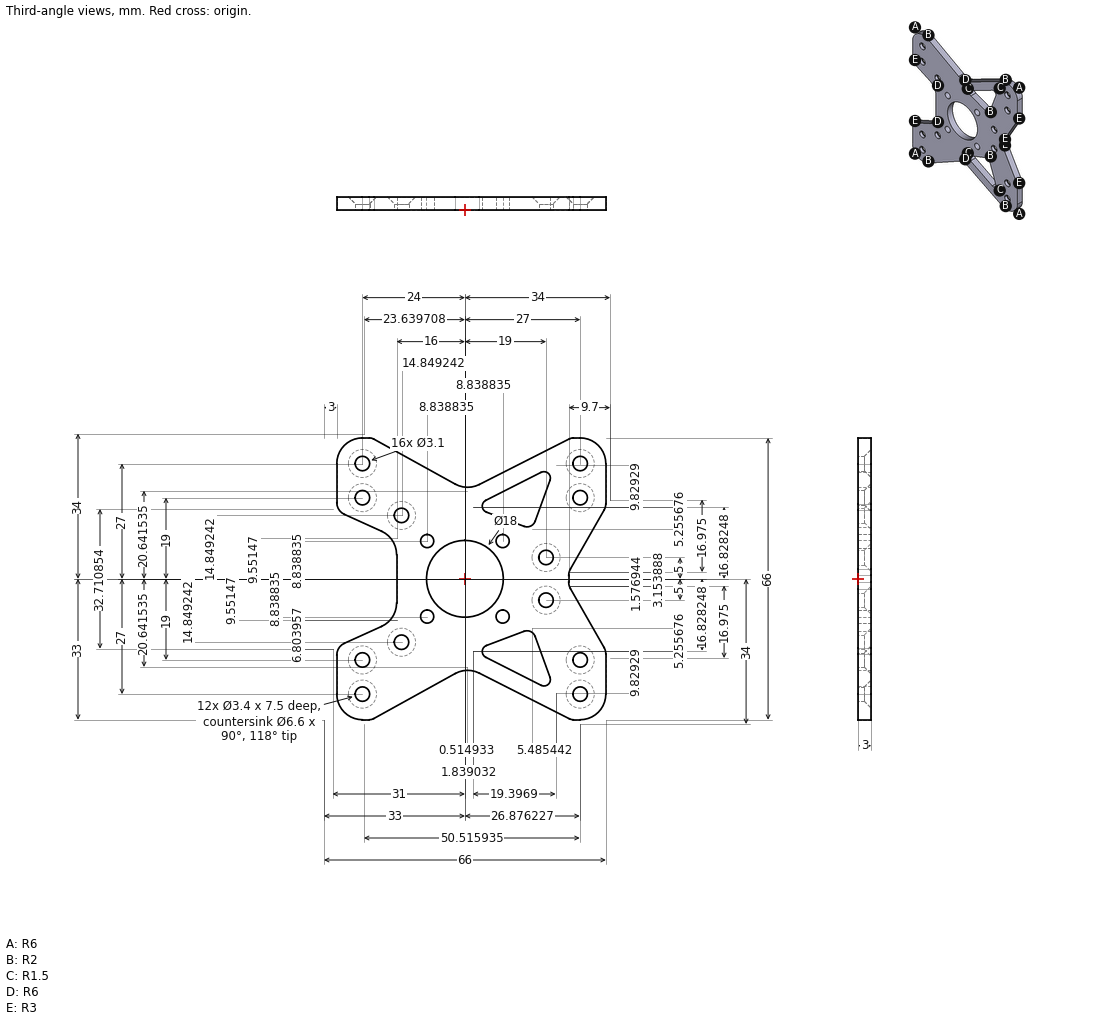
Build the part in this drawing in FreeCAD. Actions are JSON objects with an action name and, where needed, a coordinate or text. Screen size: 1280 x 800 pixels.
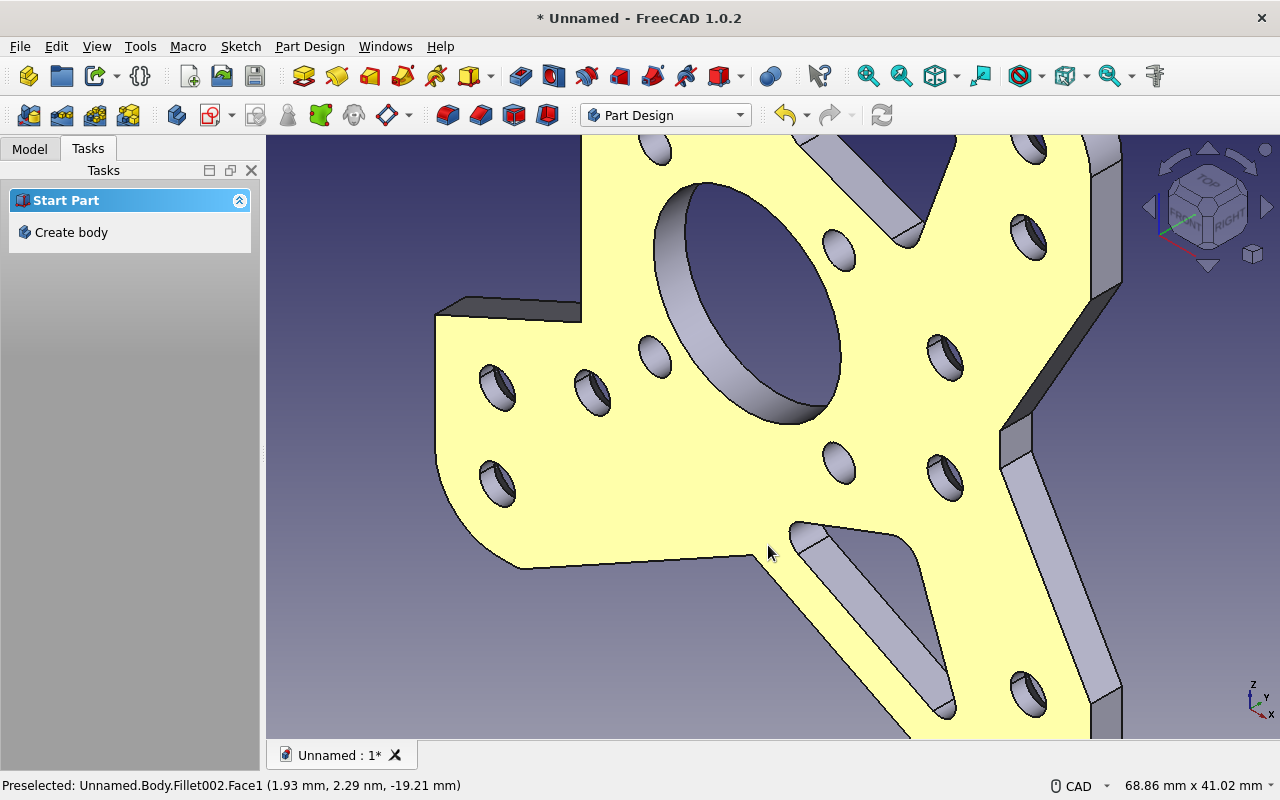
{"action": "left_click", "coordinate": [869, 76]}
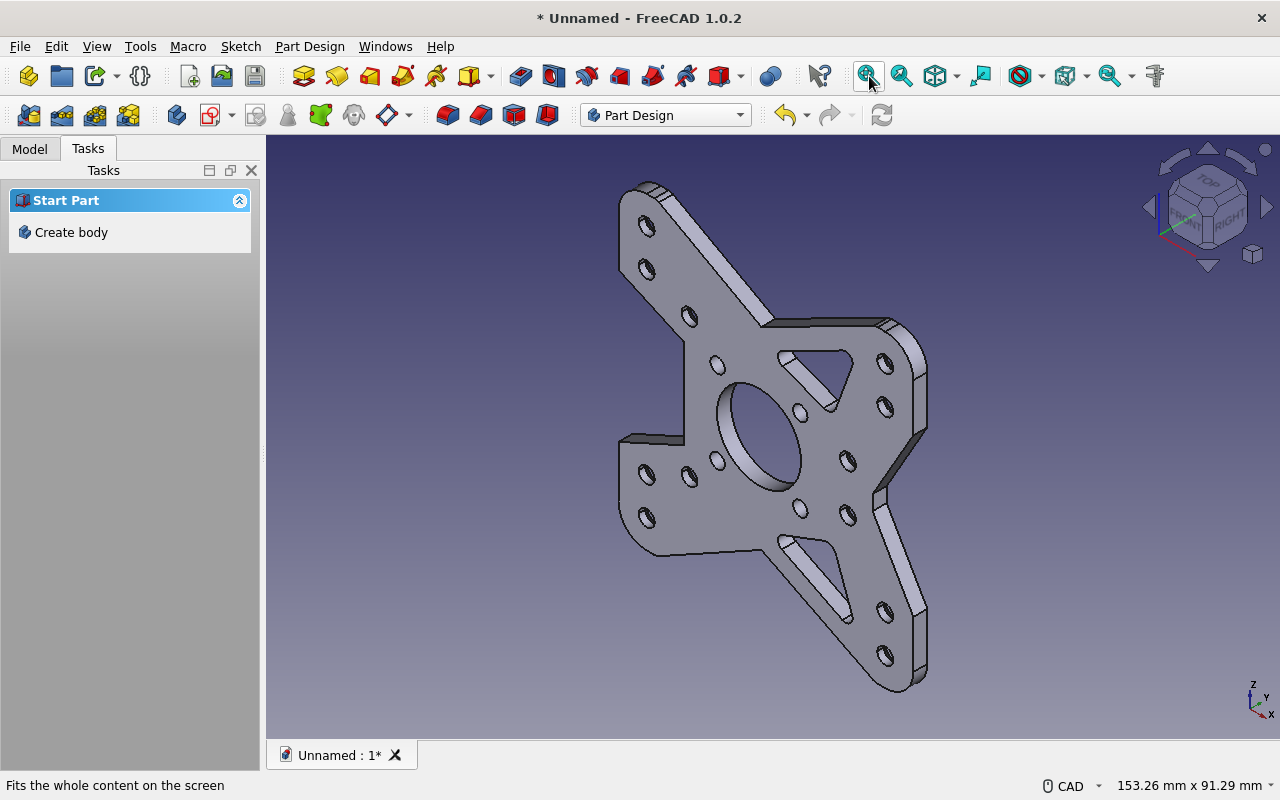
{"action": "key", "text": "2"}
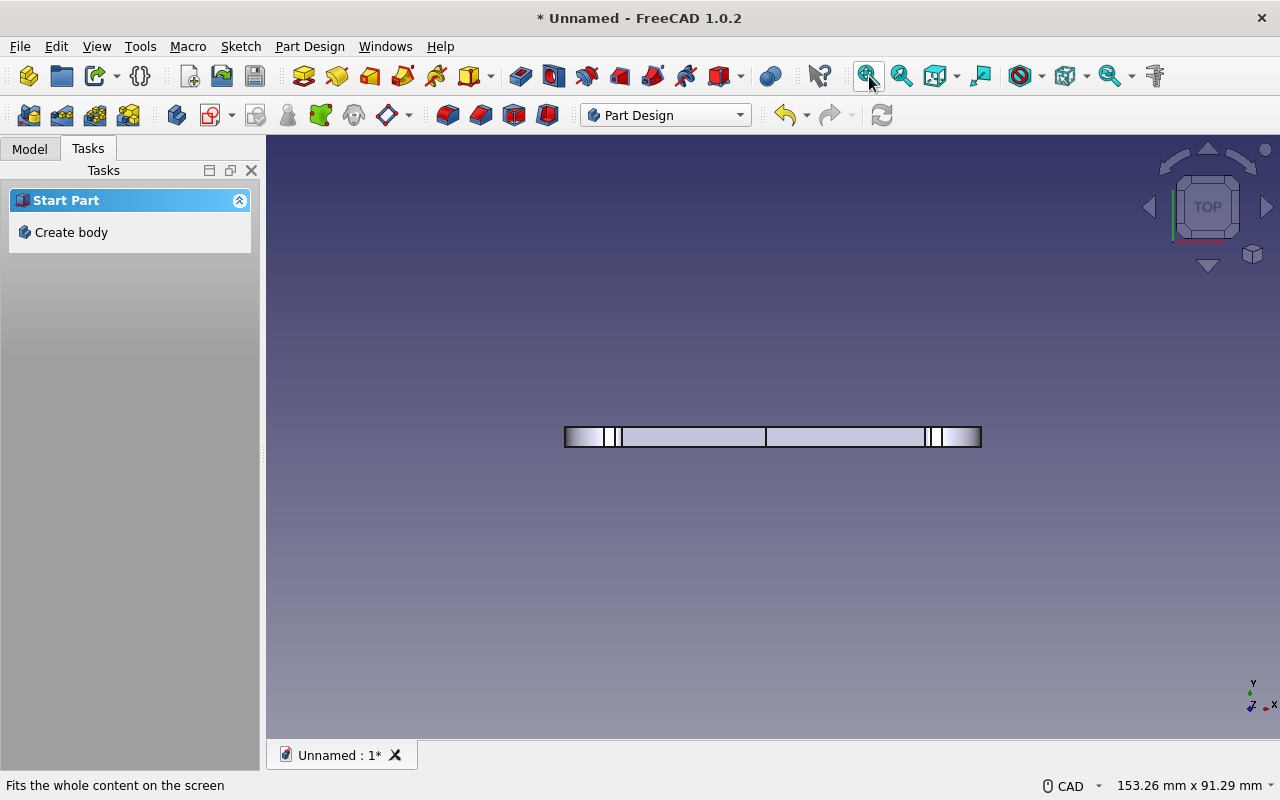
{"action": "key", "text": "v f"}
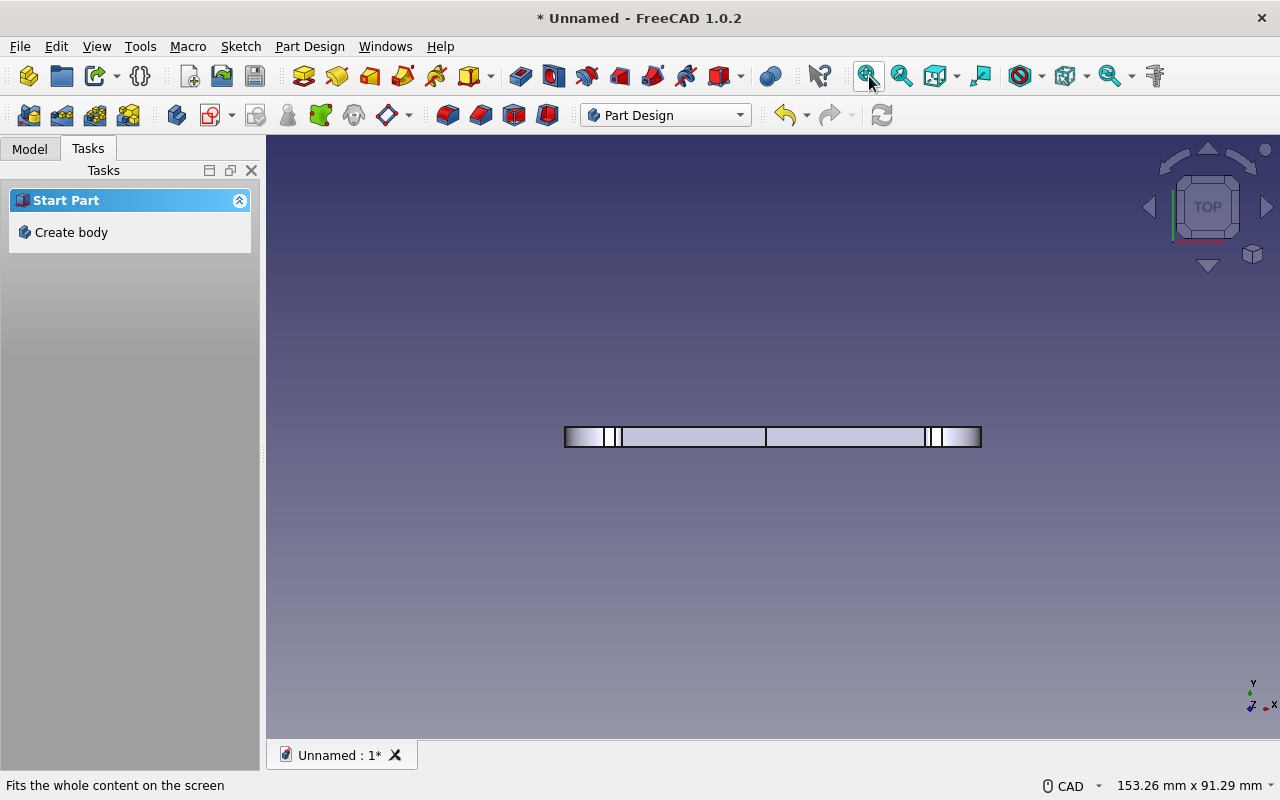
{"action": "scroll", "coordinate": [766, 436], "scroll_direction": "up", "scroll_amount": 4}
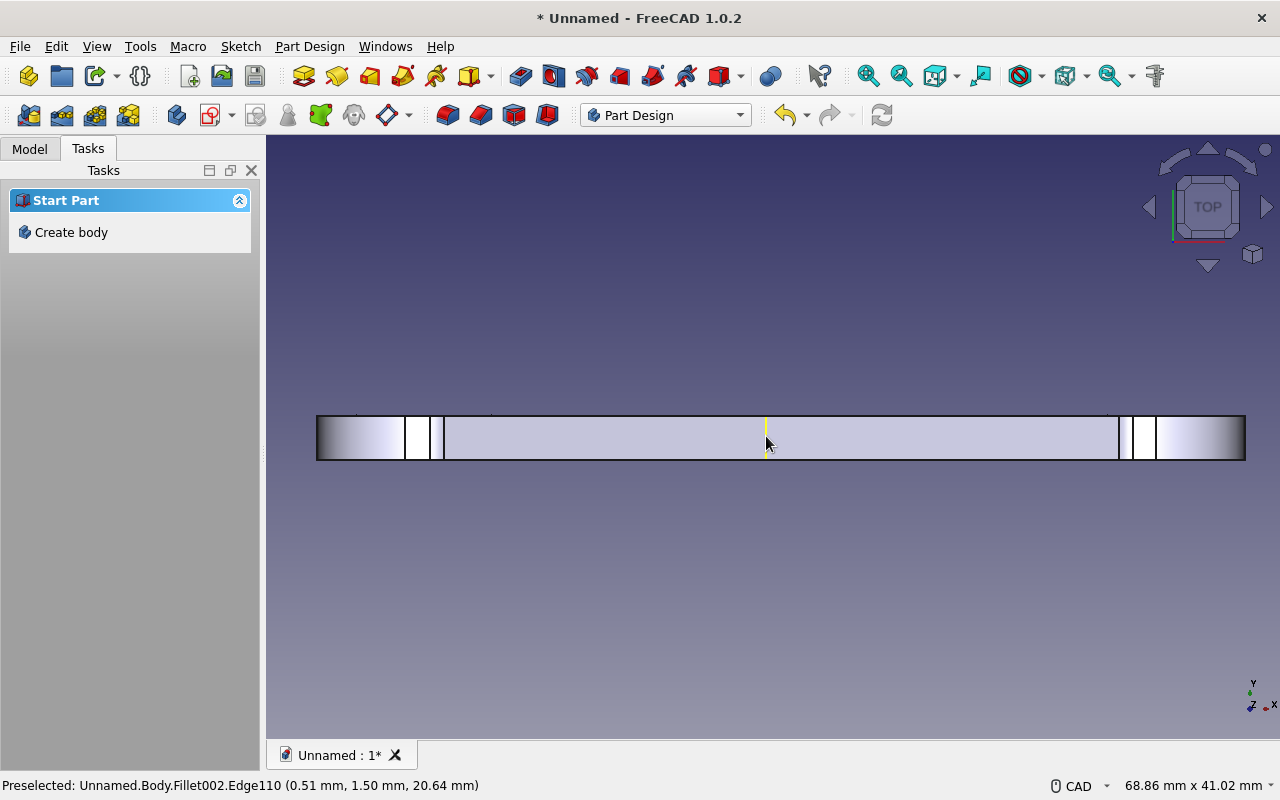
{"action": "left_click", "coordinate": [869, 76]}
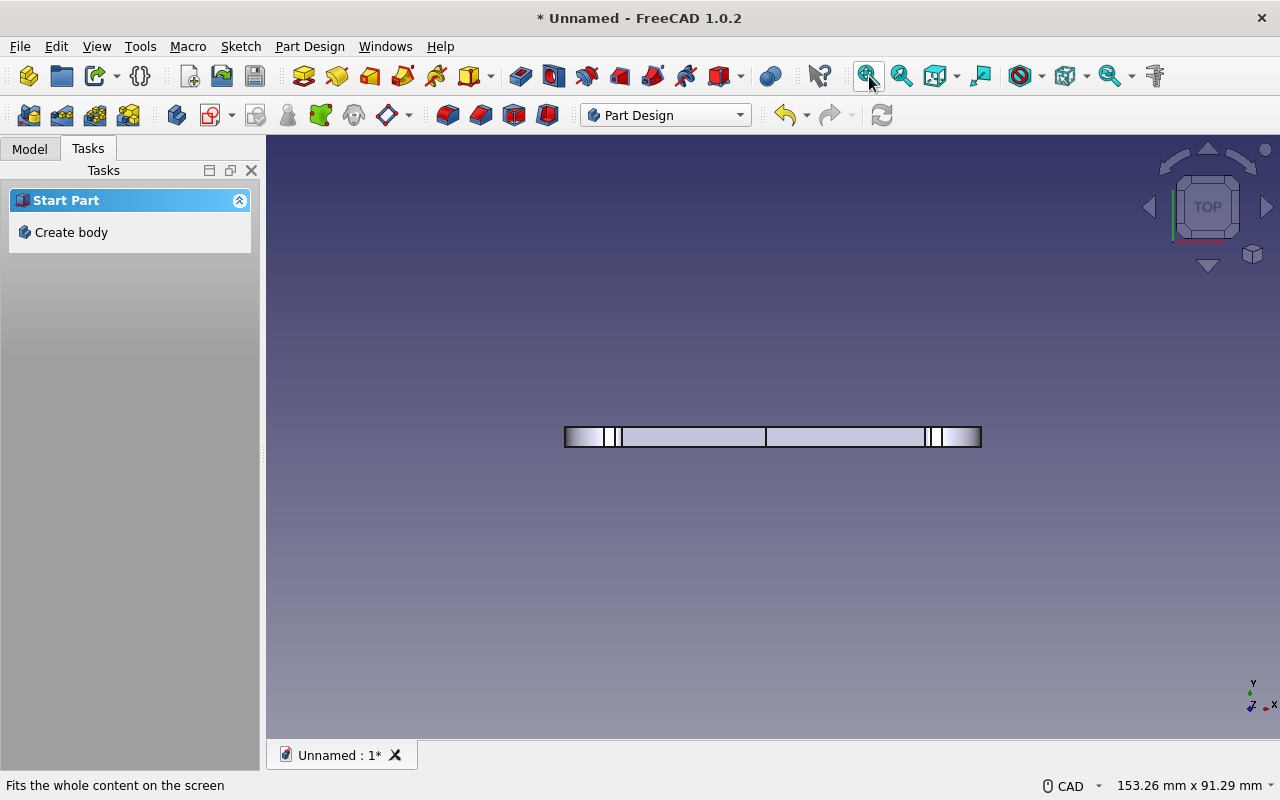
{"action": "key", "text": "0"}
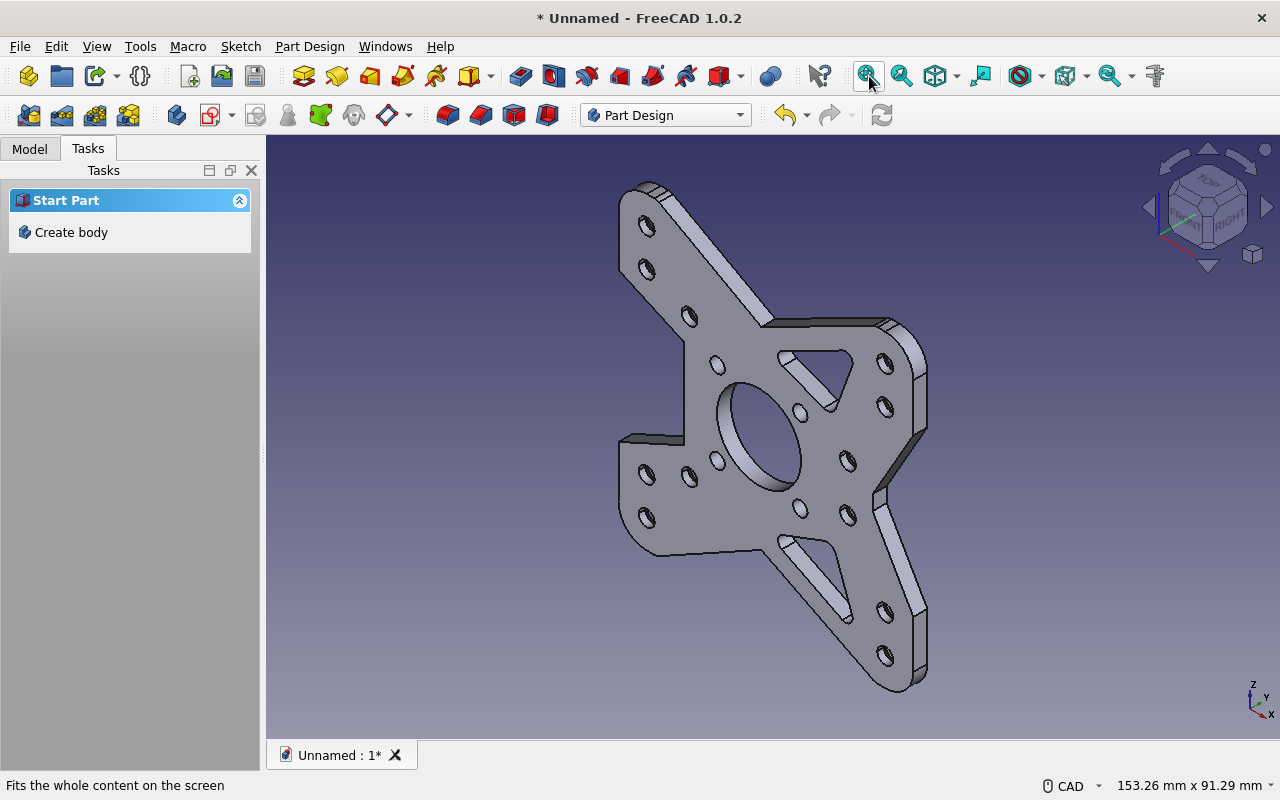
{"action": "scroll", "coordinate": [768, 545], "scroll_direction": "up", "scroll_amount": 4}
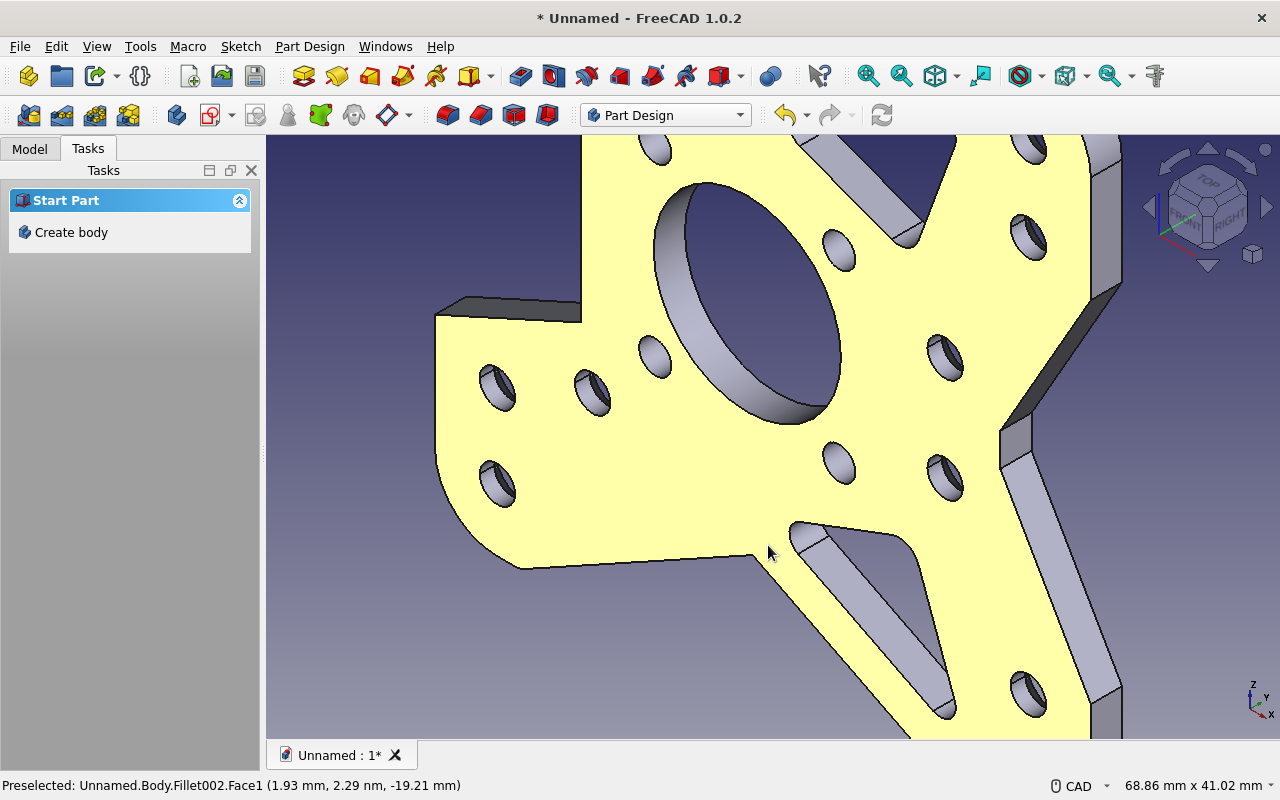
{"action": "key", "text": "v f"}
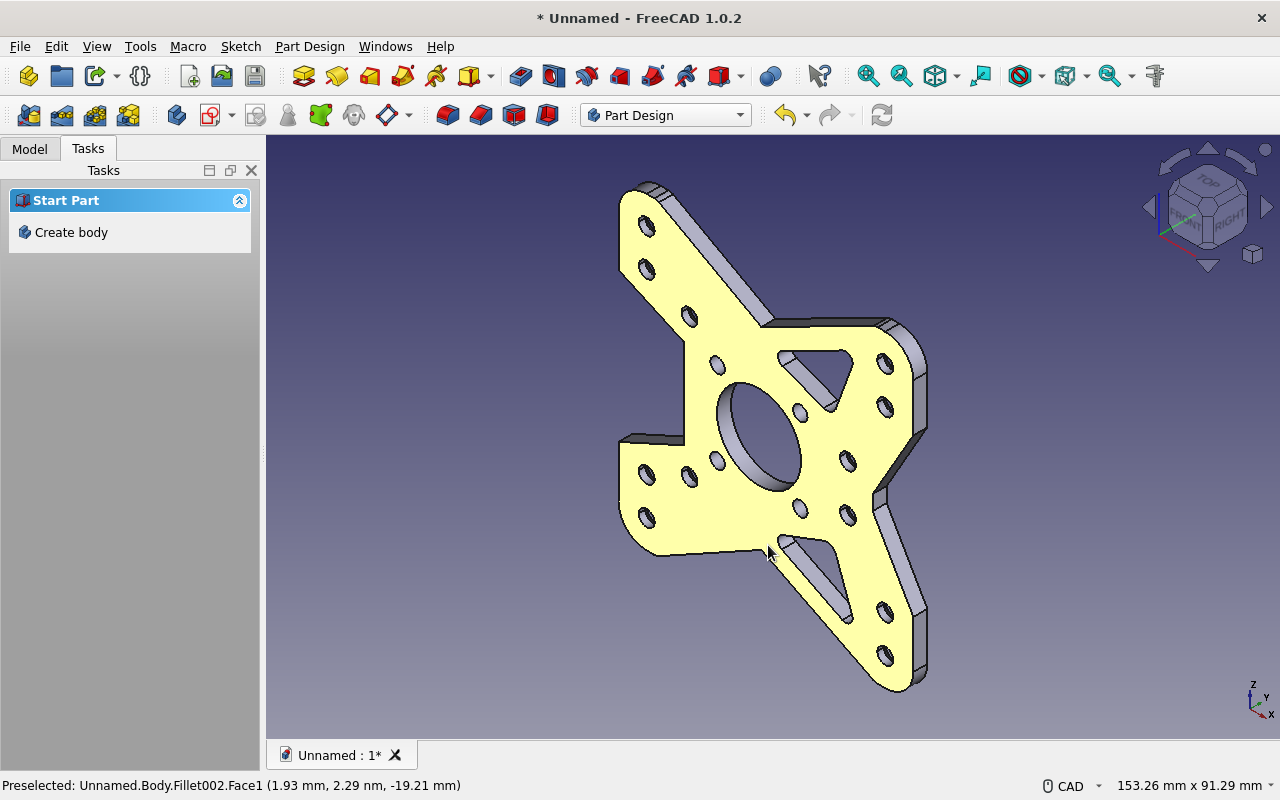
{"action": "key", "text": "1"}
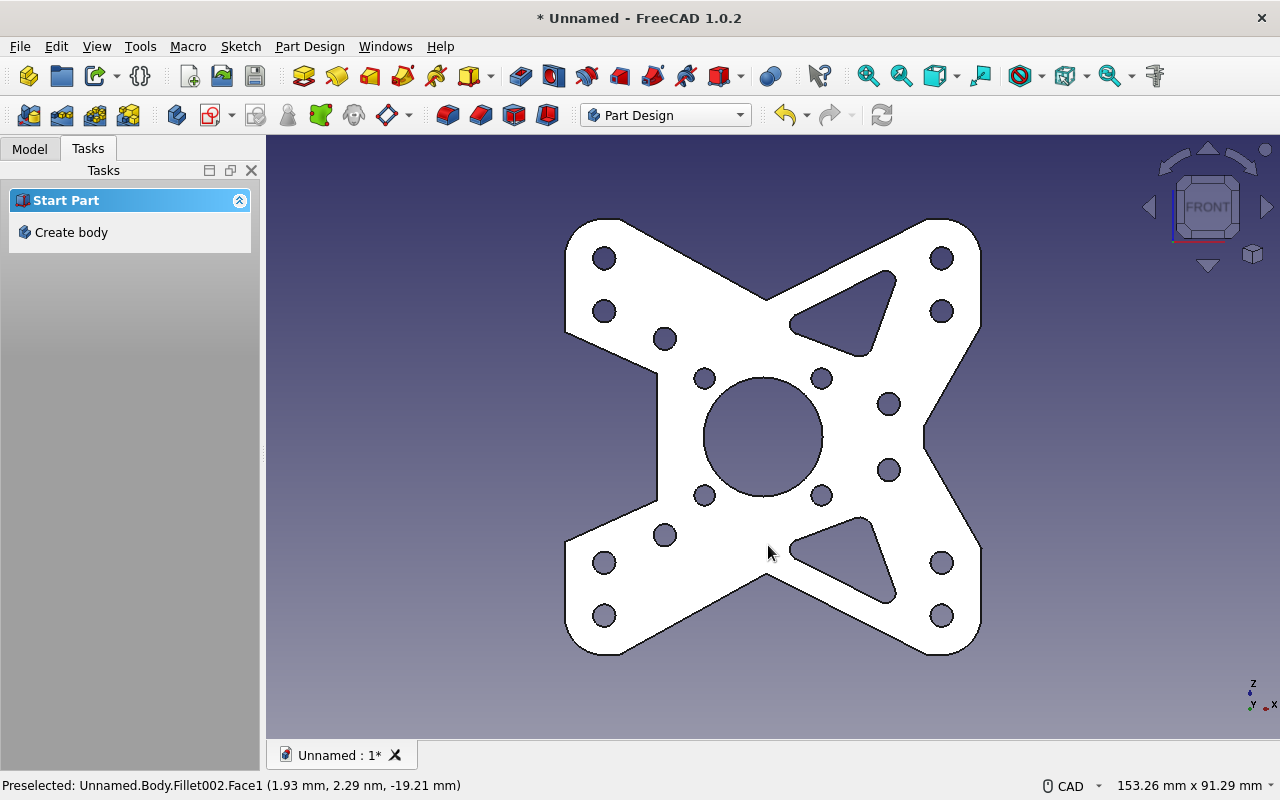
{"action": "scroll", "coordinate": [766, 573], "scroll_direction": "up", "scroll_amount": 4}